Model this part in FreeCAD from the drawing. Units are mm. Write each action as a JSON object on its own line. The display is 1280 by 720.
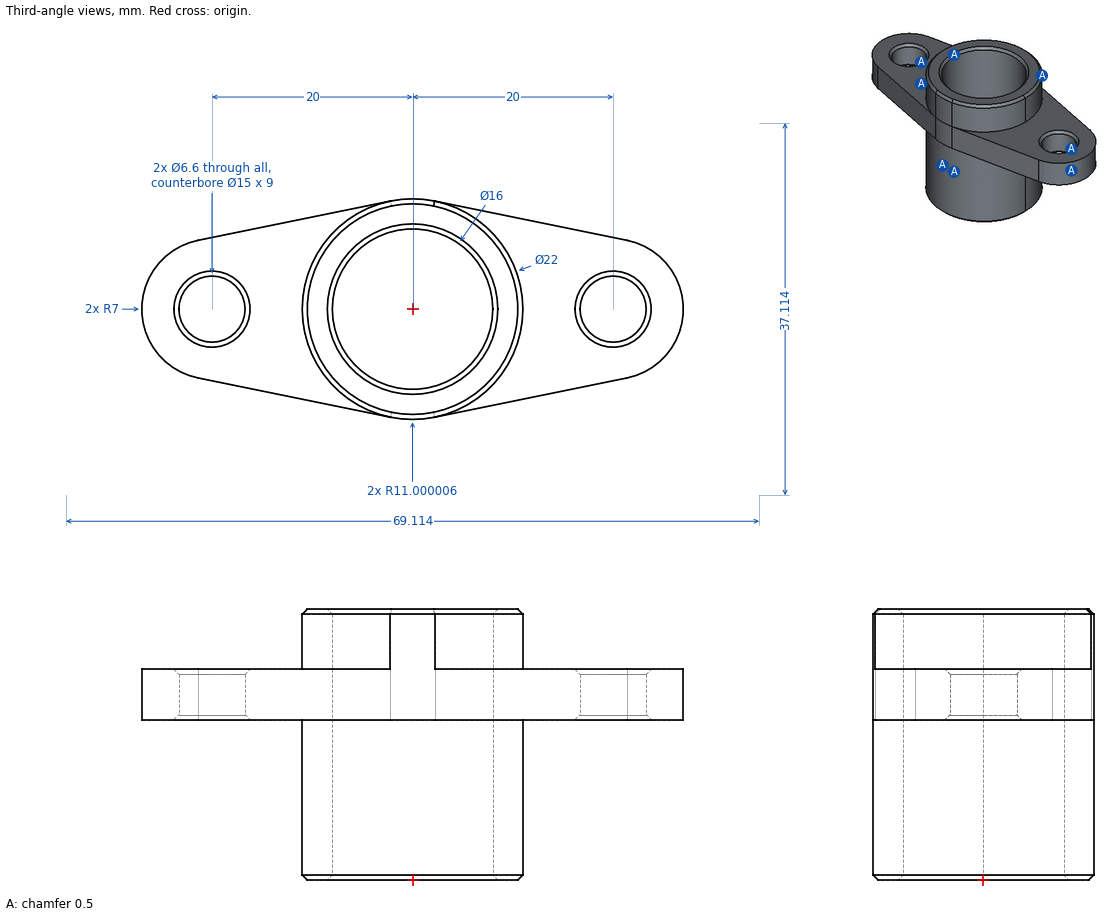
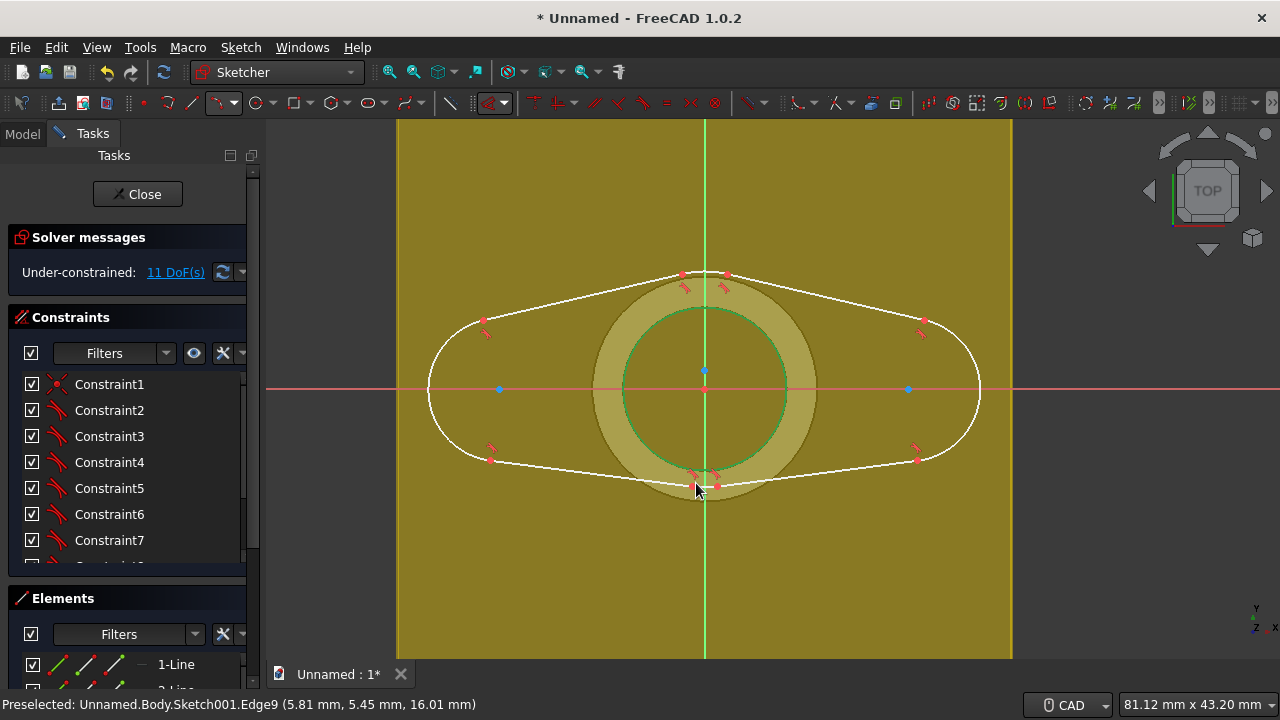
{"action": "scroll", "coordinate": [714, 272], "scroll_direction": "up", "scroll_amount": 3}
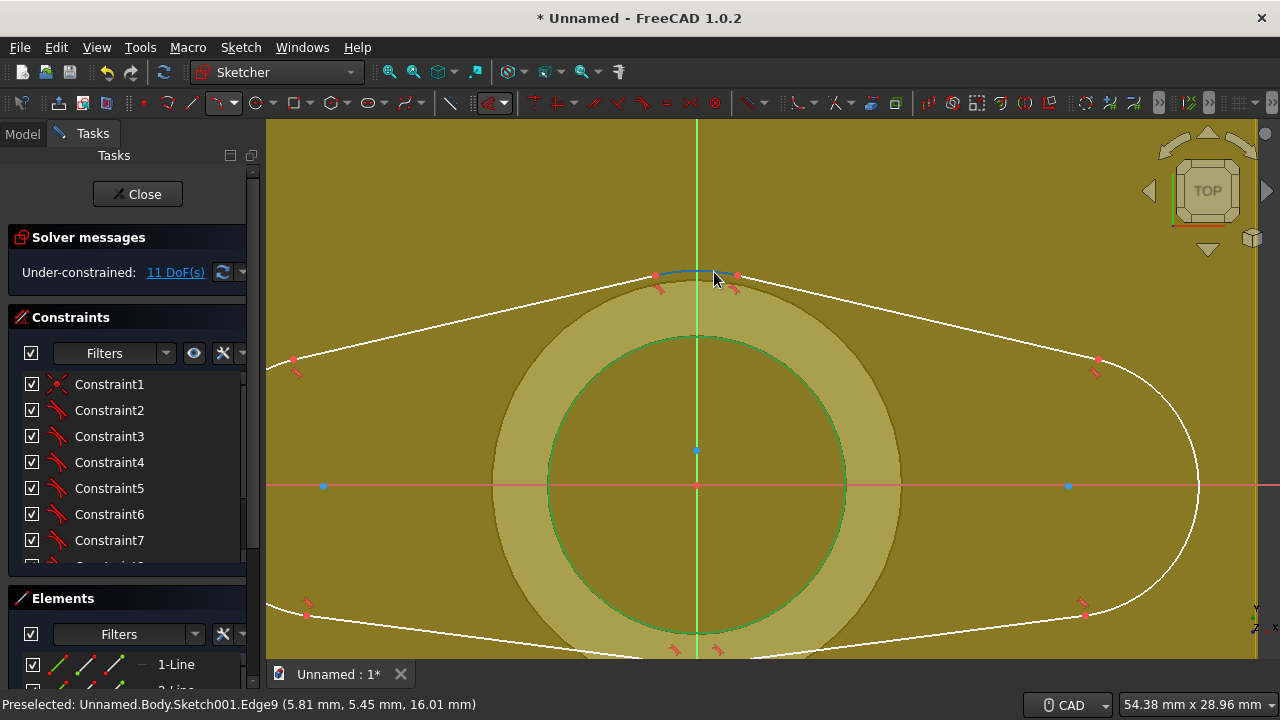
{"action": "left_click", "coordinate": [713, 272]}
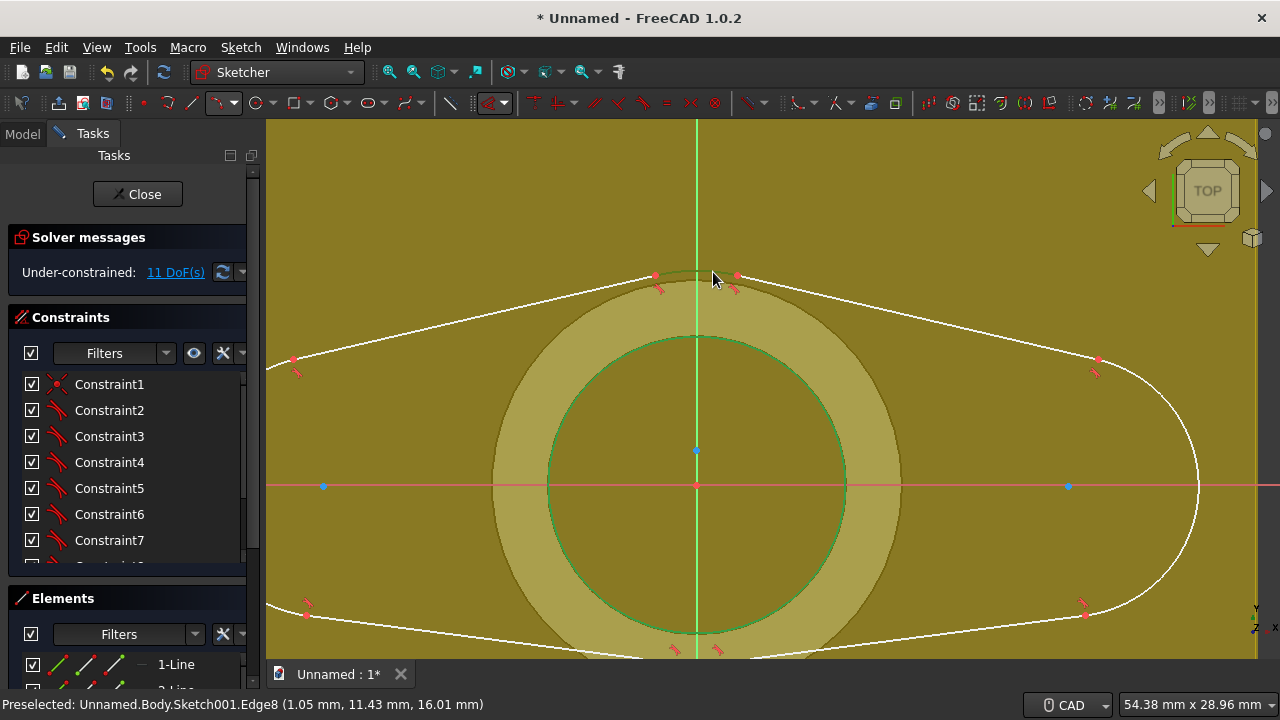
{"action": "left_click", "coordinate": [534, 104]}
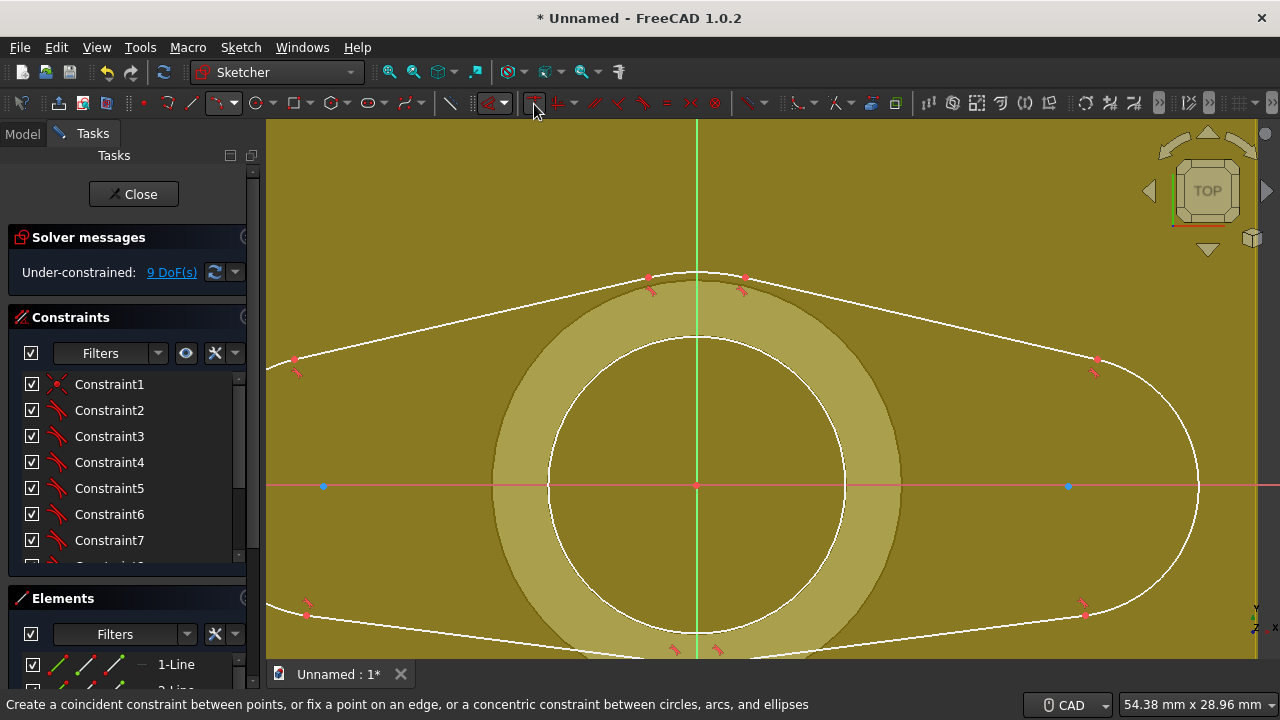
{"action": "scroll", "coordinate": [714, 272], "scroll_direction": "down", "scroll_amount": 3}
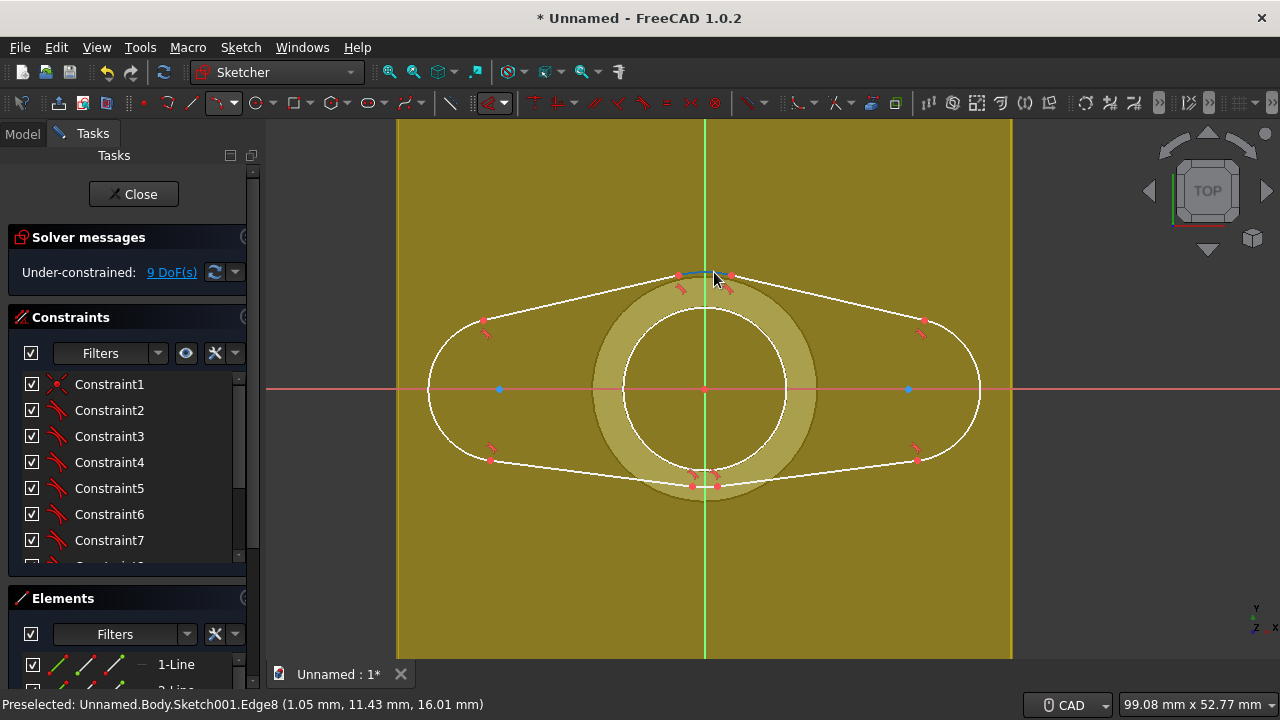
{"action": "left_click", "coordinate": [437, 355]}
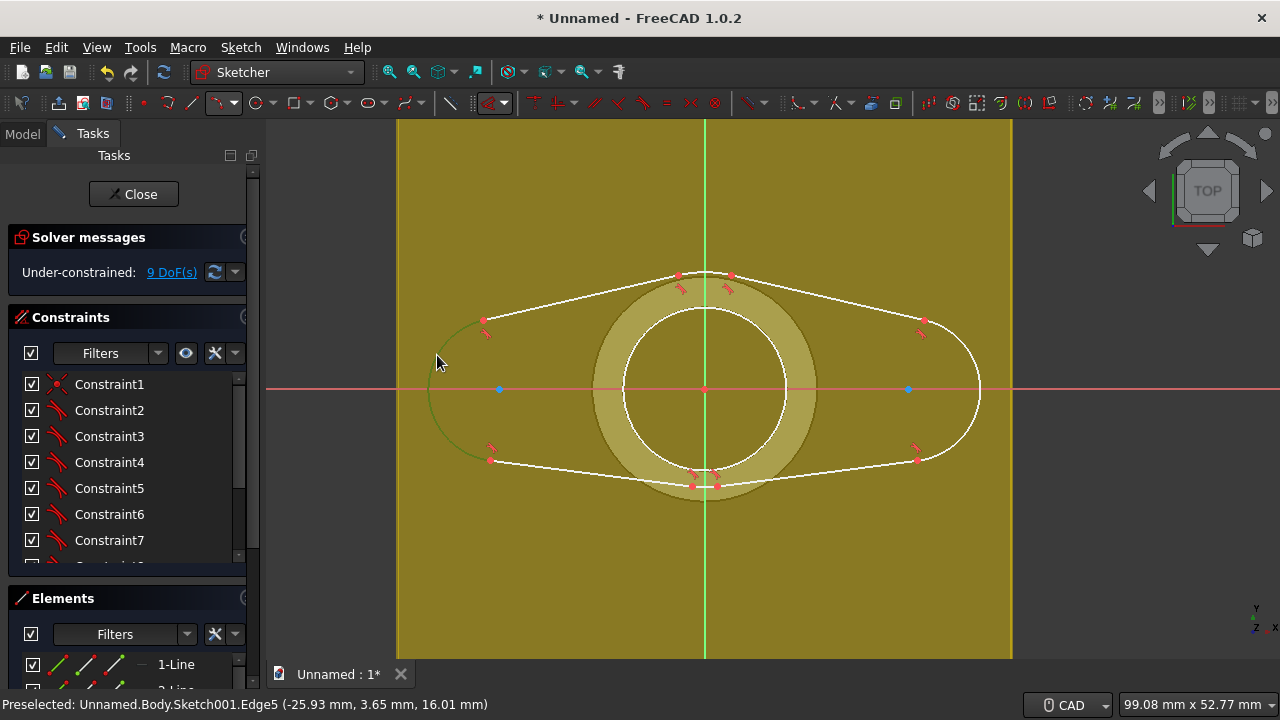
{"action": "left_click", "coordinate": [967, 431]}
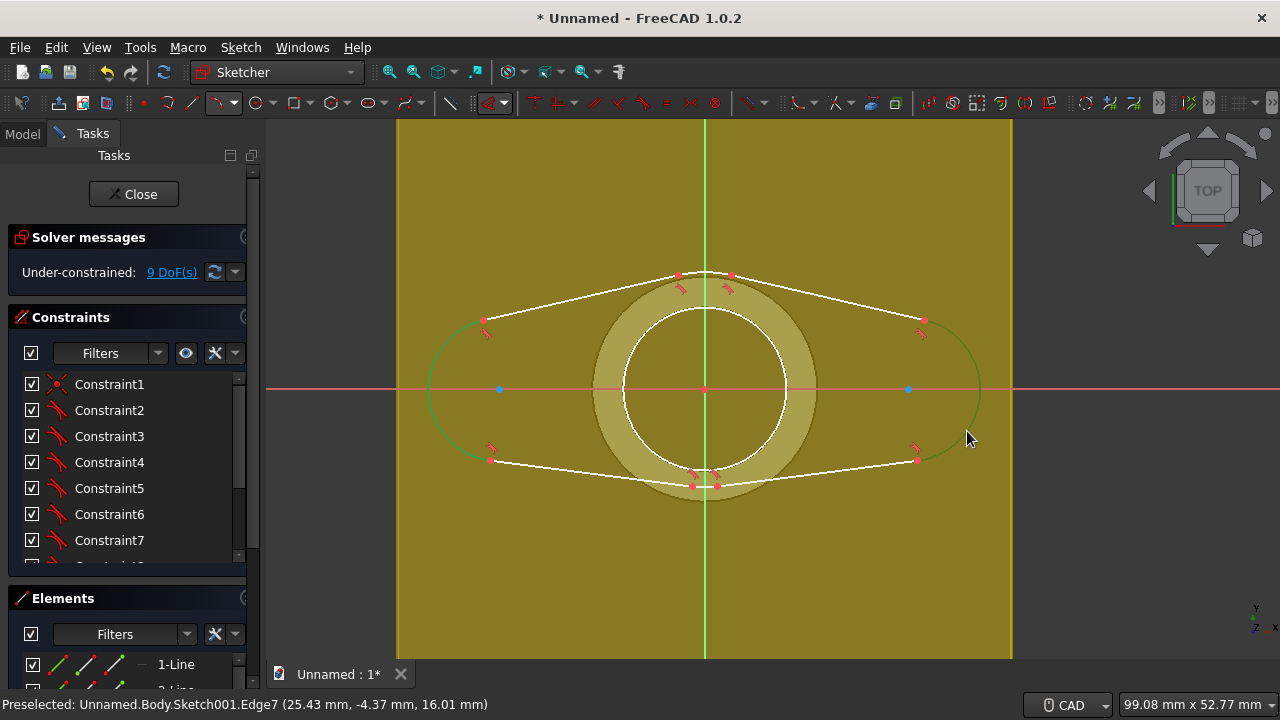
{"action": "left_click", "coordinate": [668, 104]}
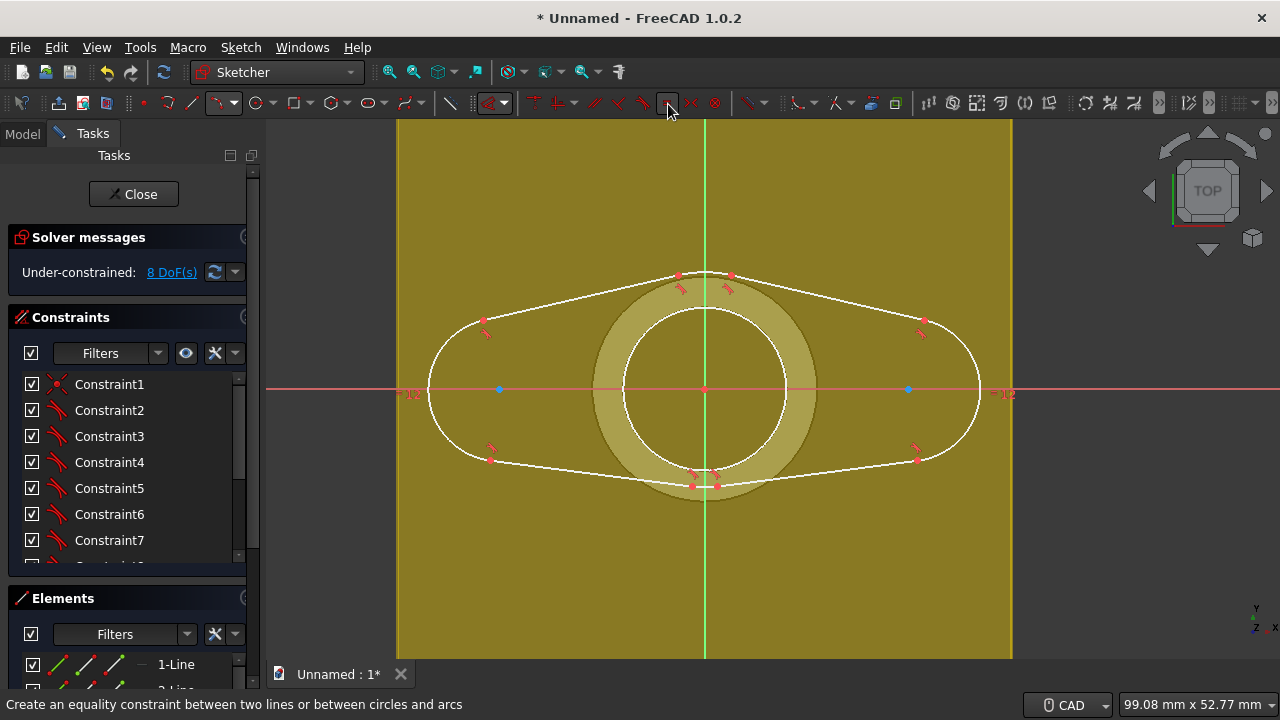
{"action": "left_click", "coordinate": [705, 487]}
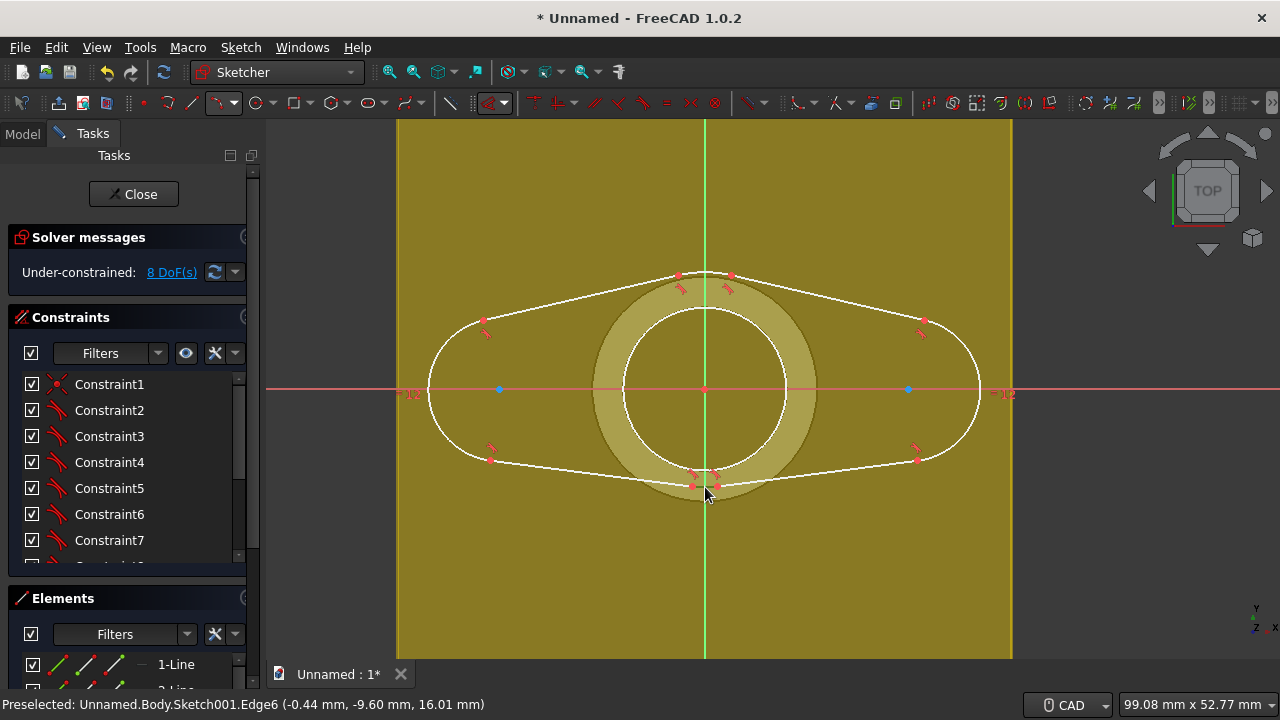
{"action": "scroll", "coordinate": [716, 273], "scroll_direction": "up", "scroll_amount": 2}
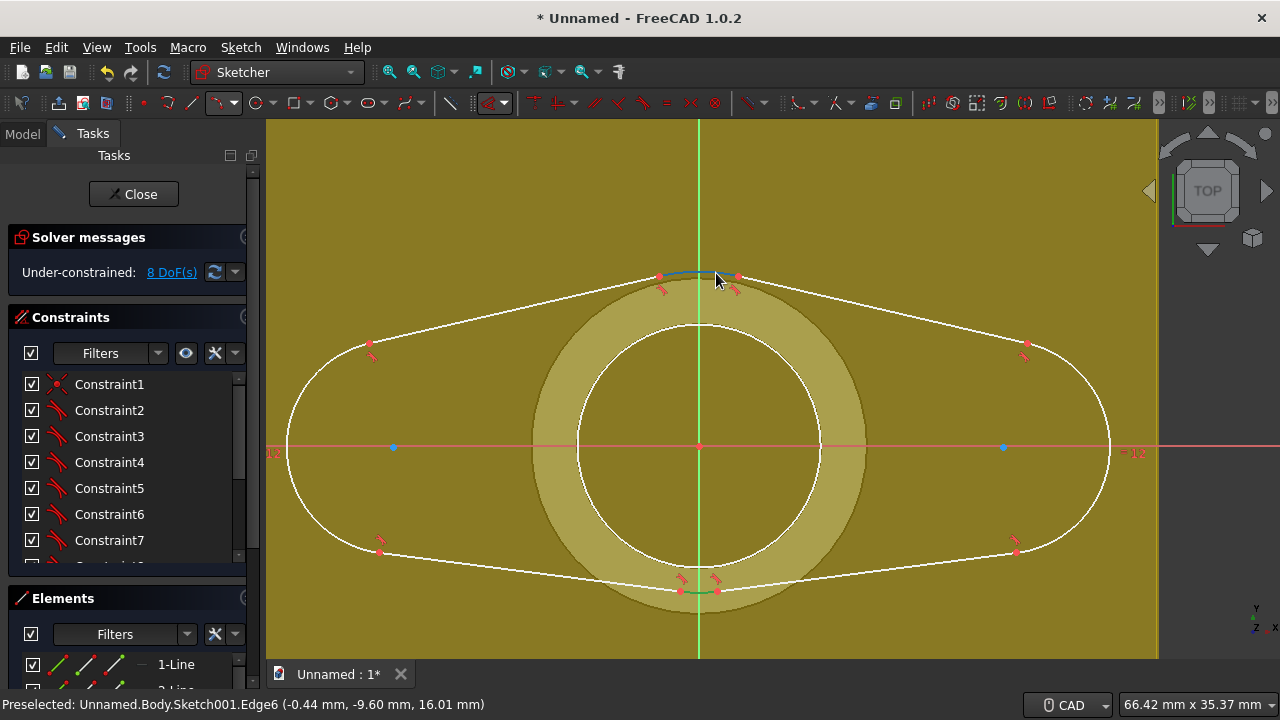
{"action": "left_click", "coordinate": [715, 272]}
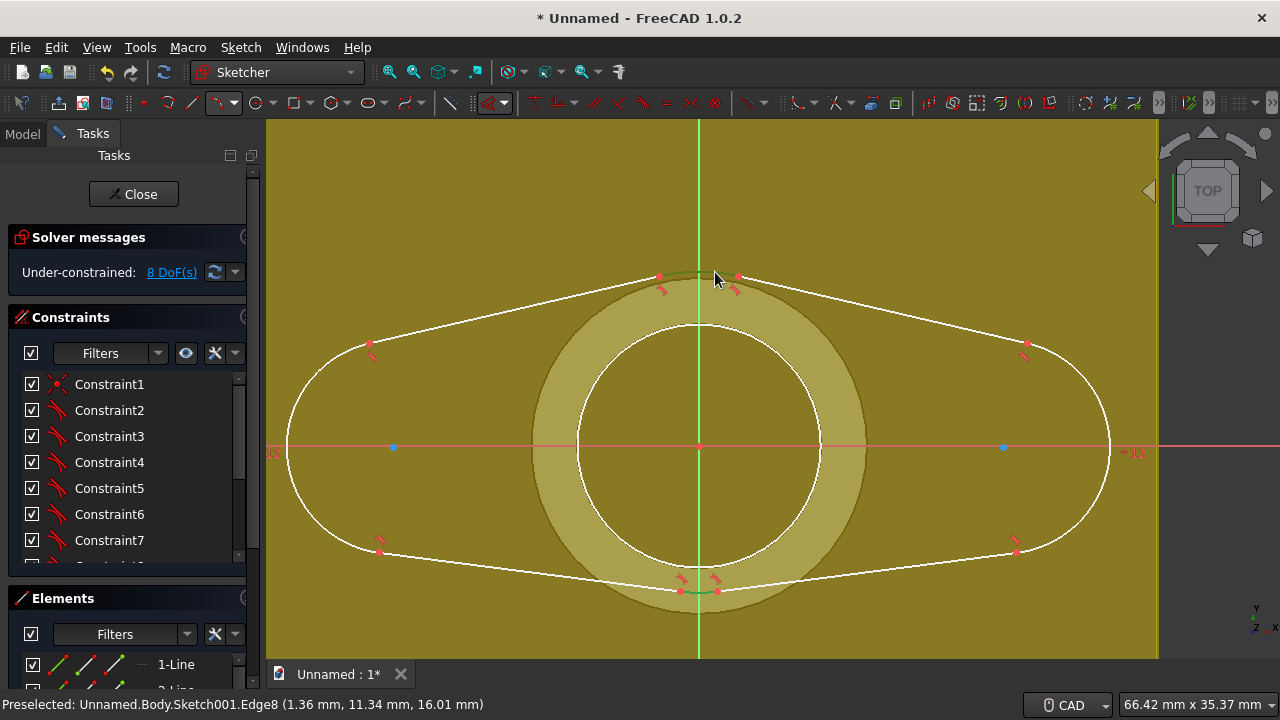
{"action": "left_click", "coordinate": [668, 104]}